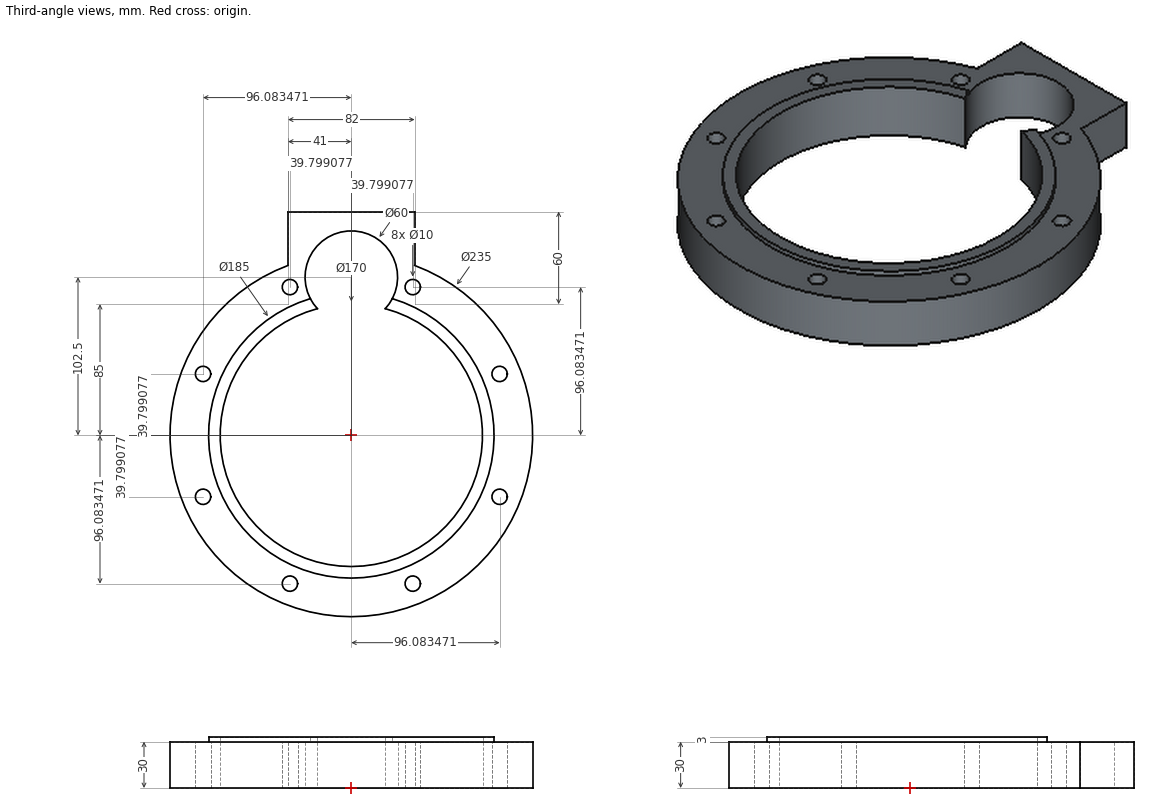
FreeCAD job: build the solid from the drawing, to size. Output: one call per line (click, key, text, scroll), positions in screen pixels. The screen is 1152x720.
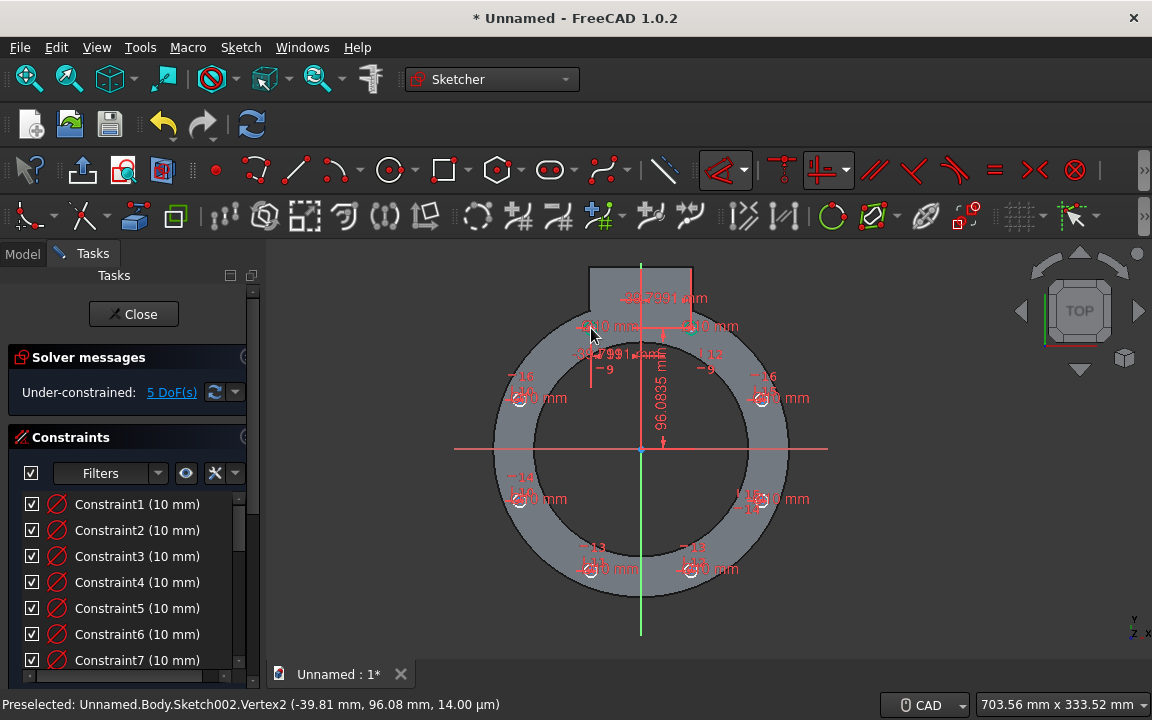
click(520, 400)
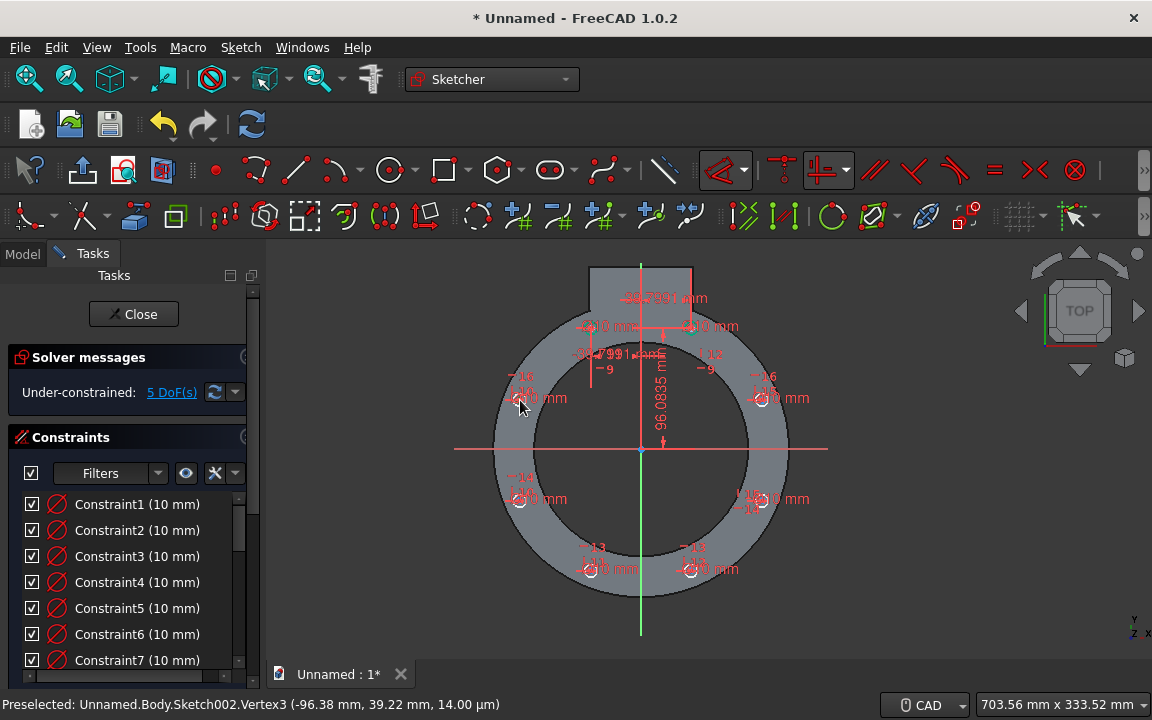
click(746, 170)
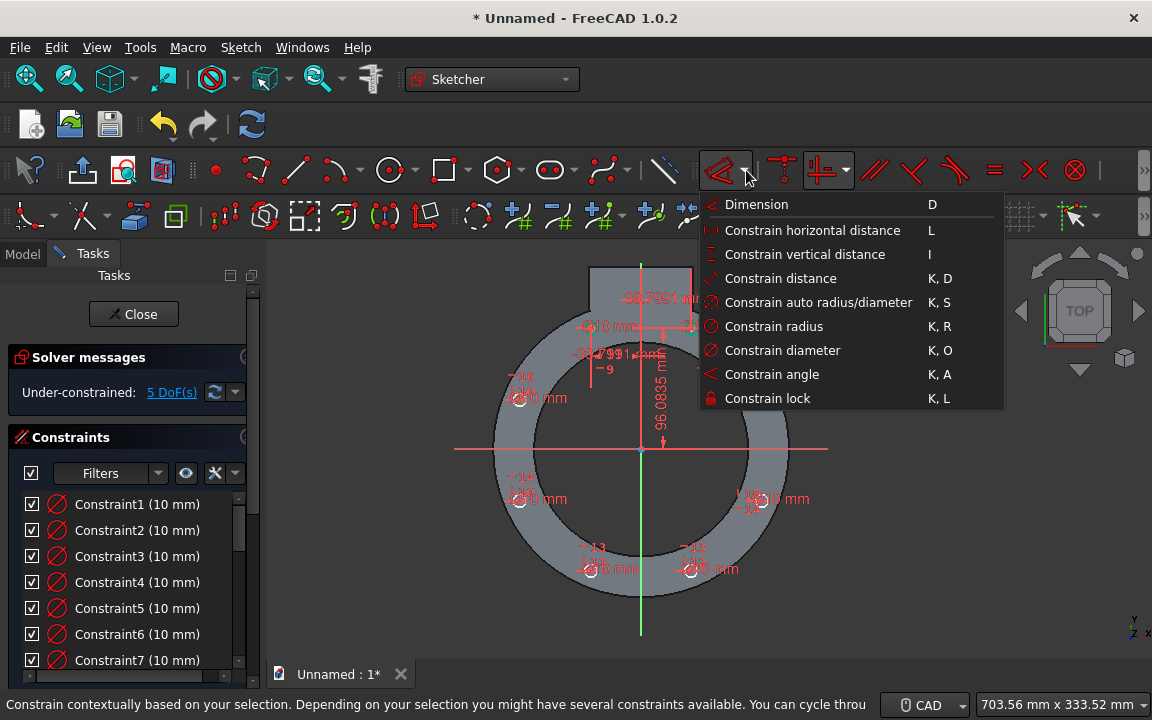
click(852, 230)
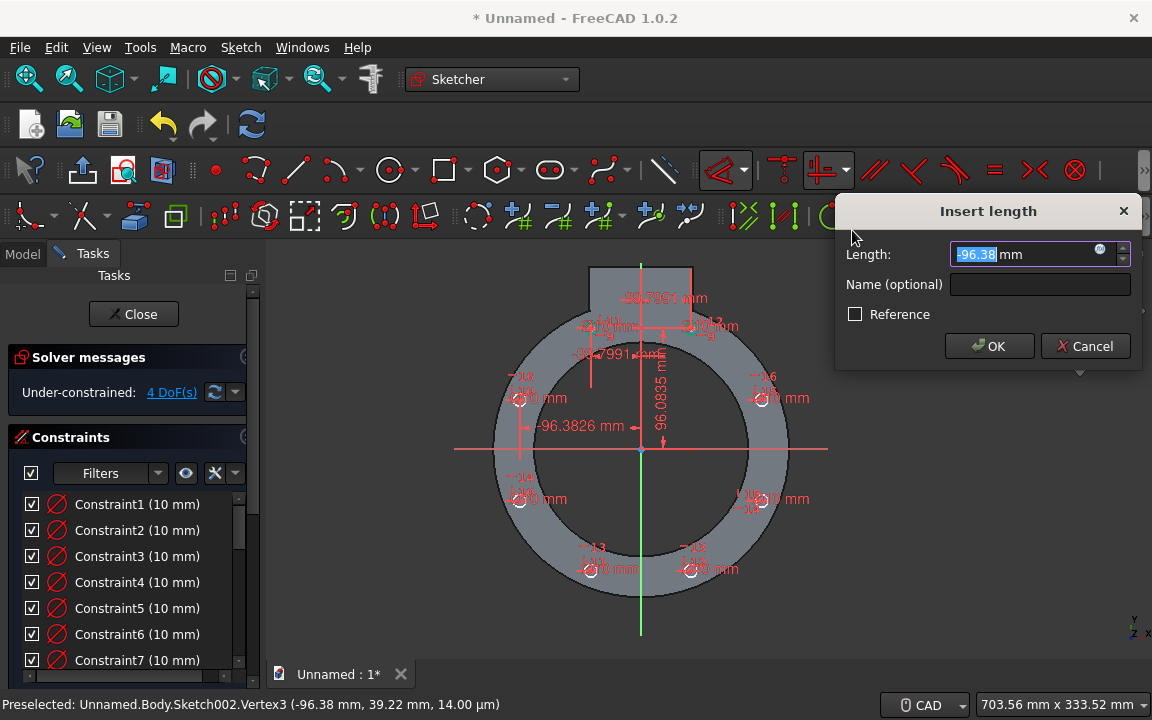
text(-96.083471)
key(Return)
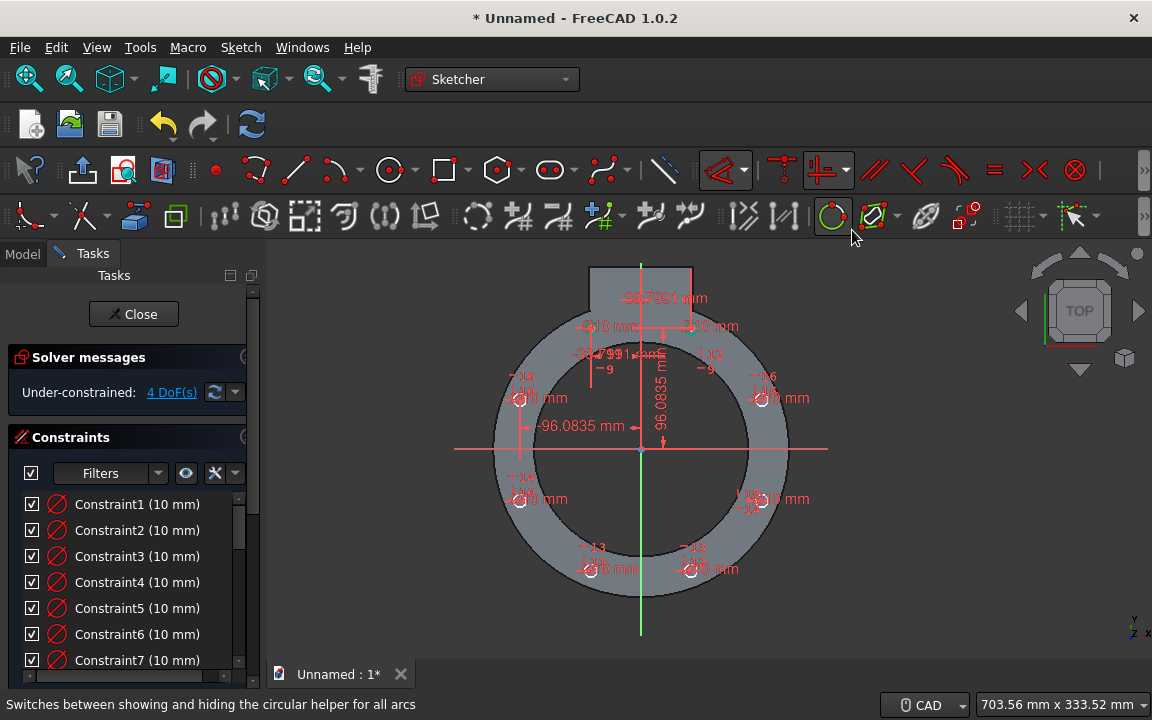
click(520, 400)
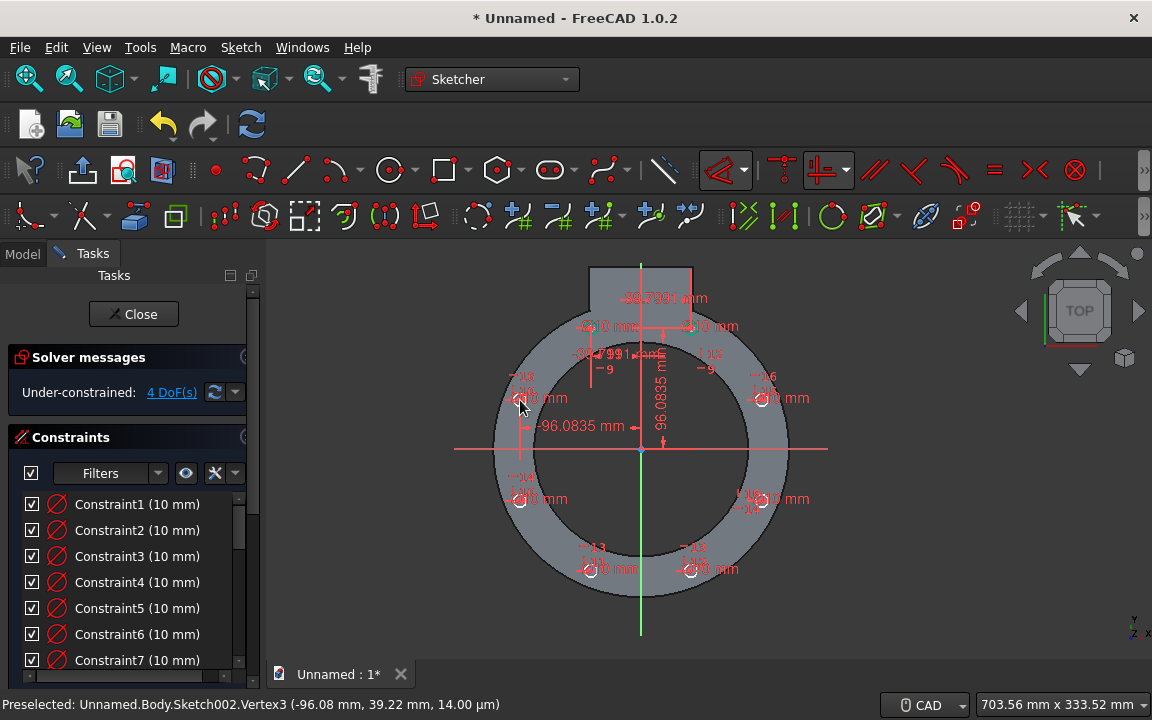
key(i)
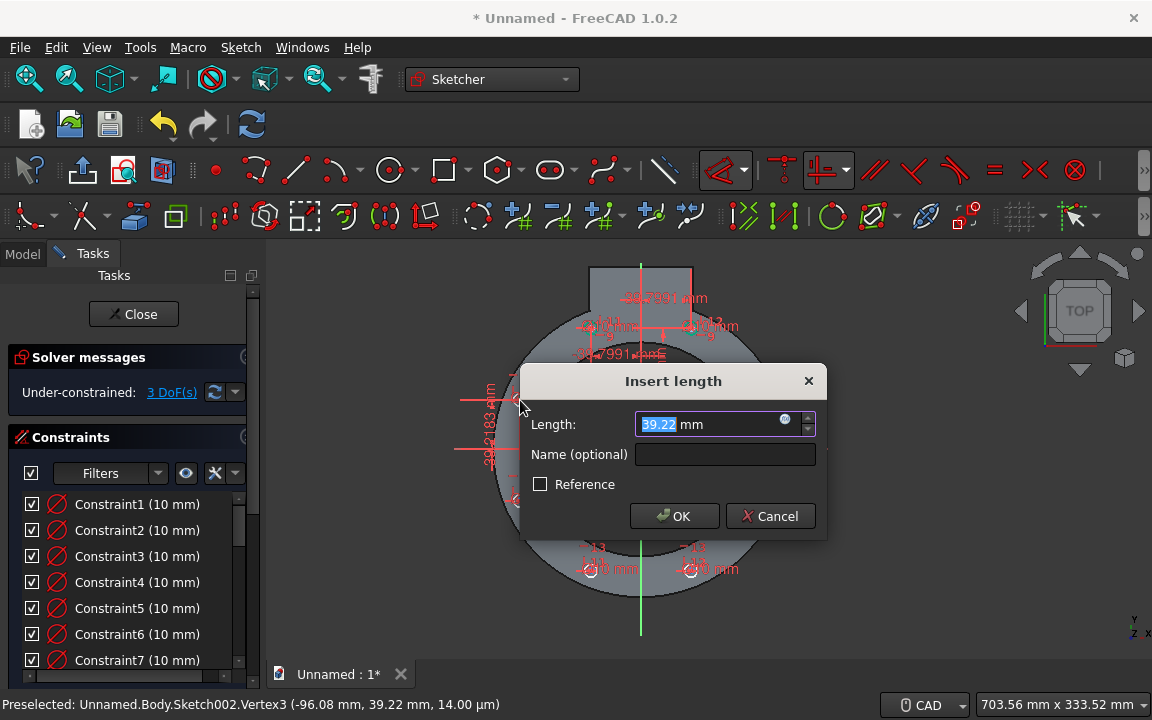
text(39.799077)
key(Return)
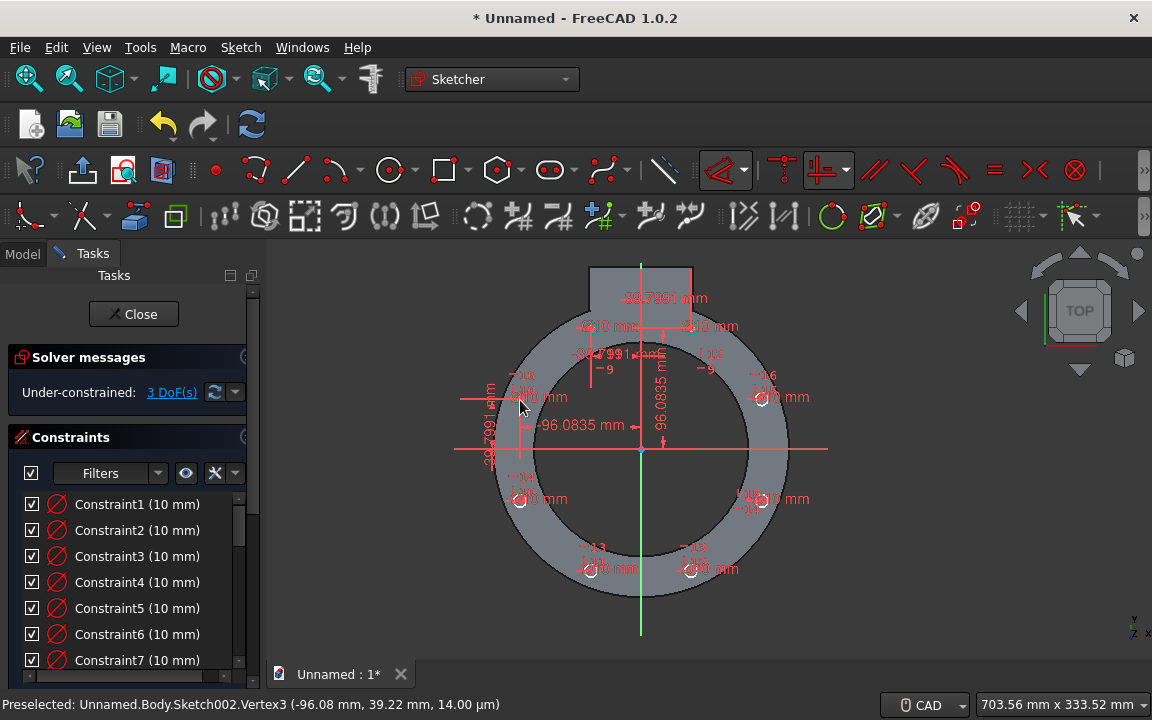
click(520, 501)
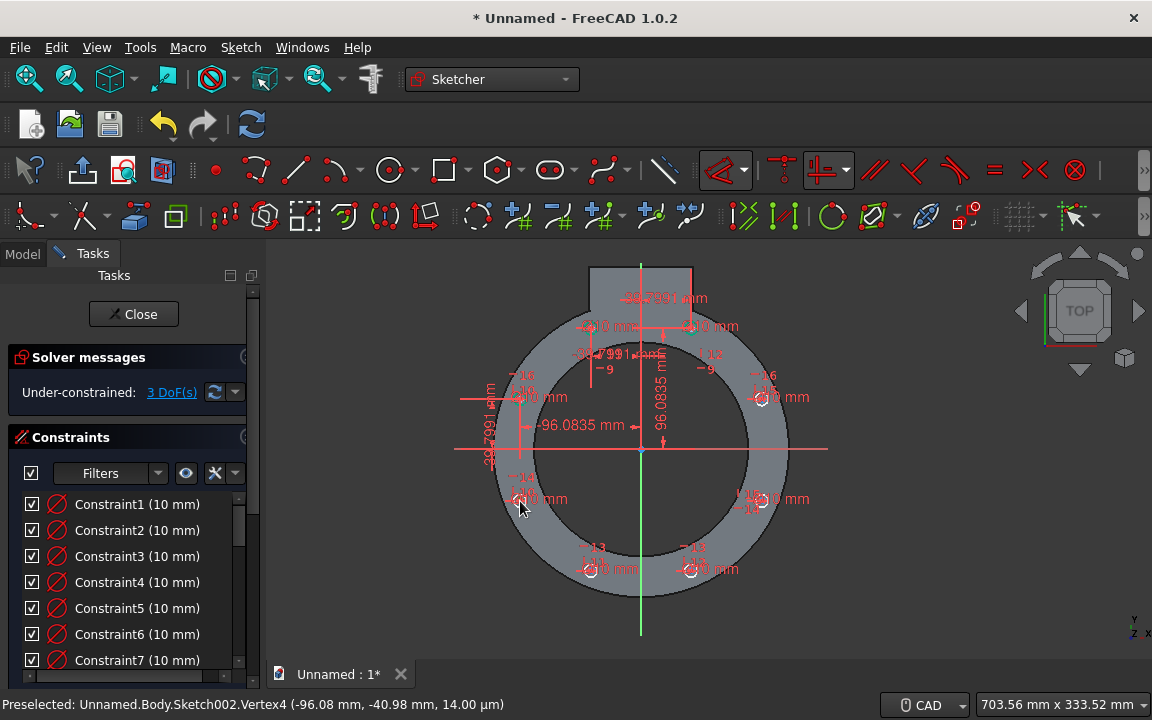
key(i)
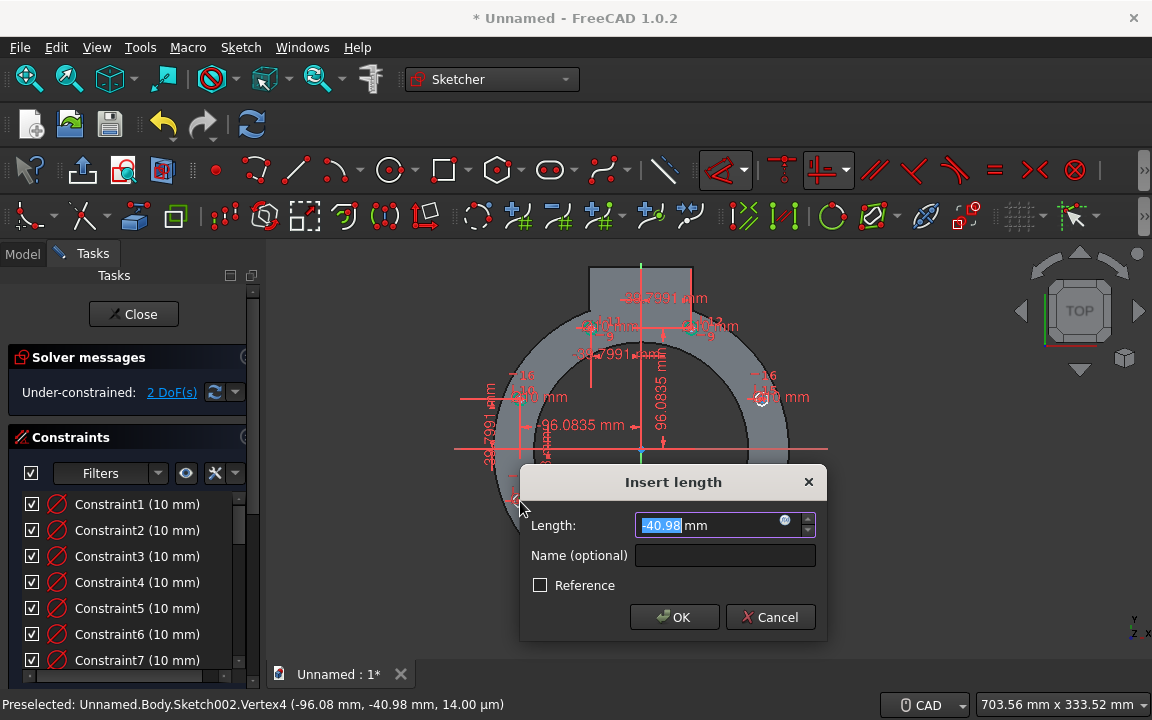
text(-39.799077)
key(Return)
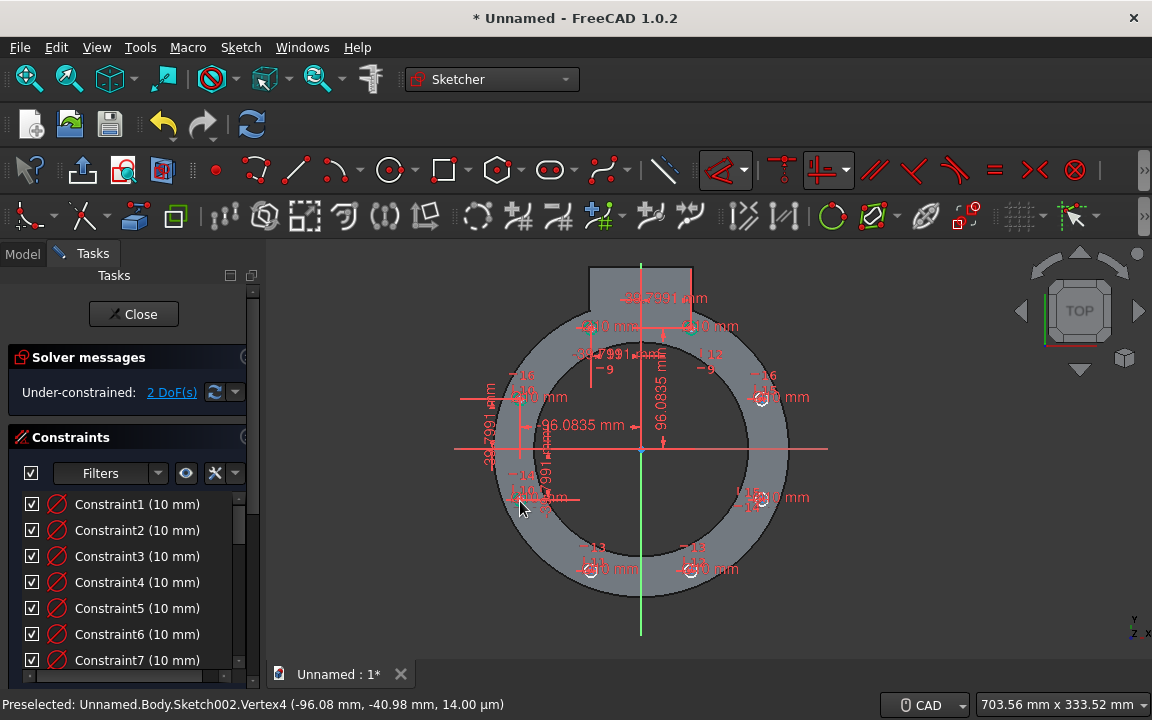
click(591, 571)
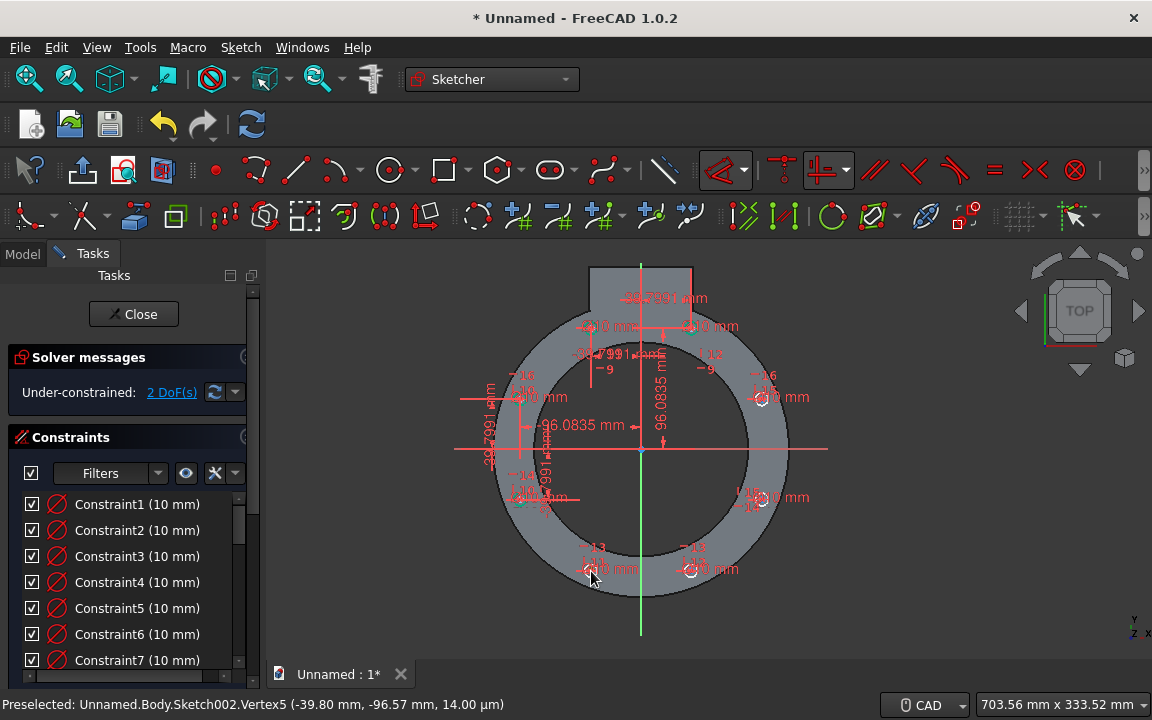
key(i)